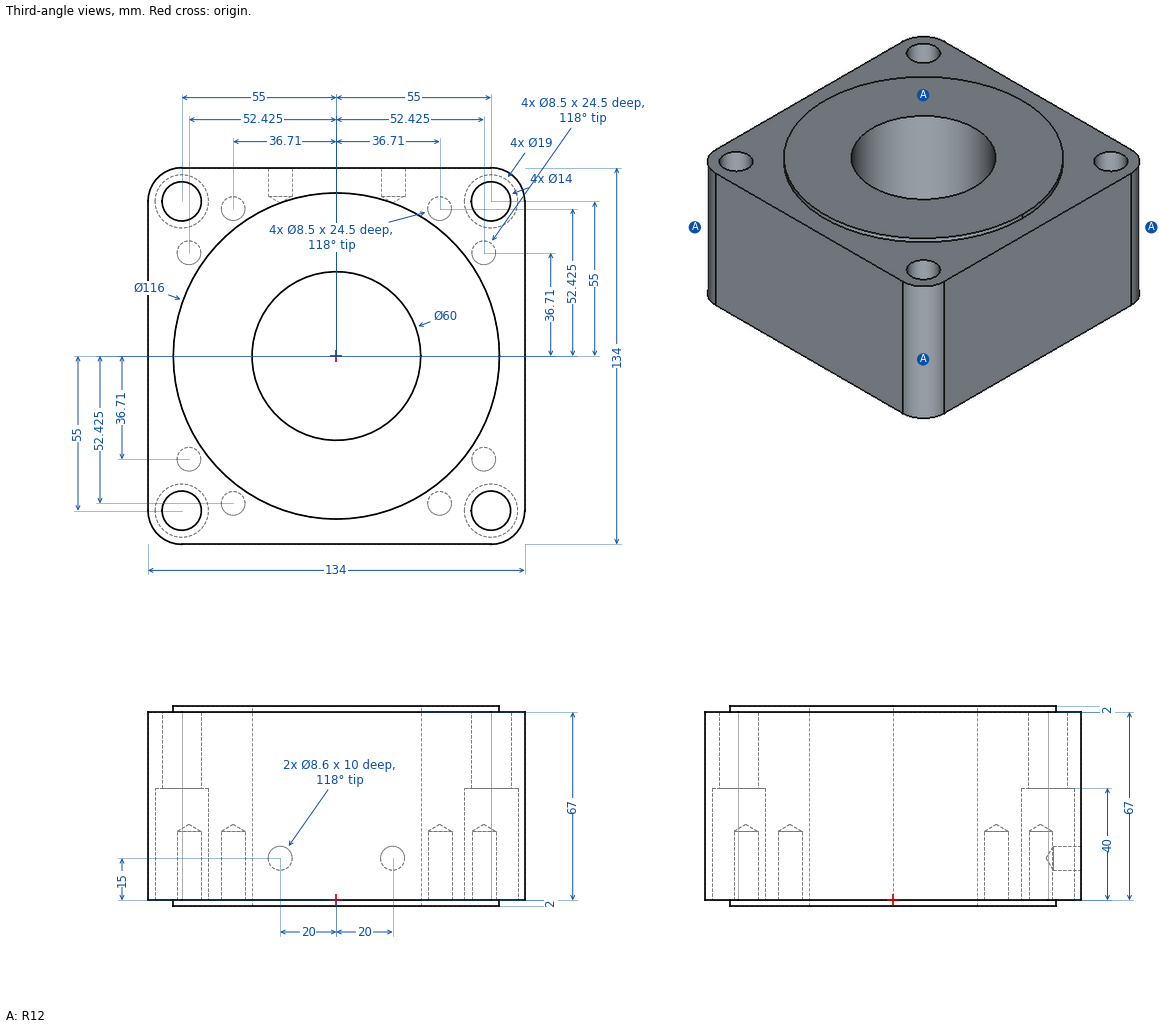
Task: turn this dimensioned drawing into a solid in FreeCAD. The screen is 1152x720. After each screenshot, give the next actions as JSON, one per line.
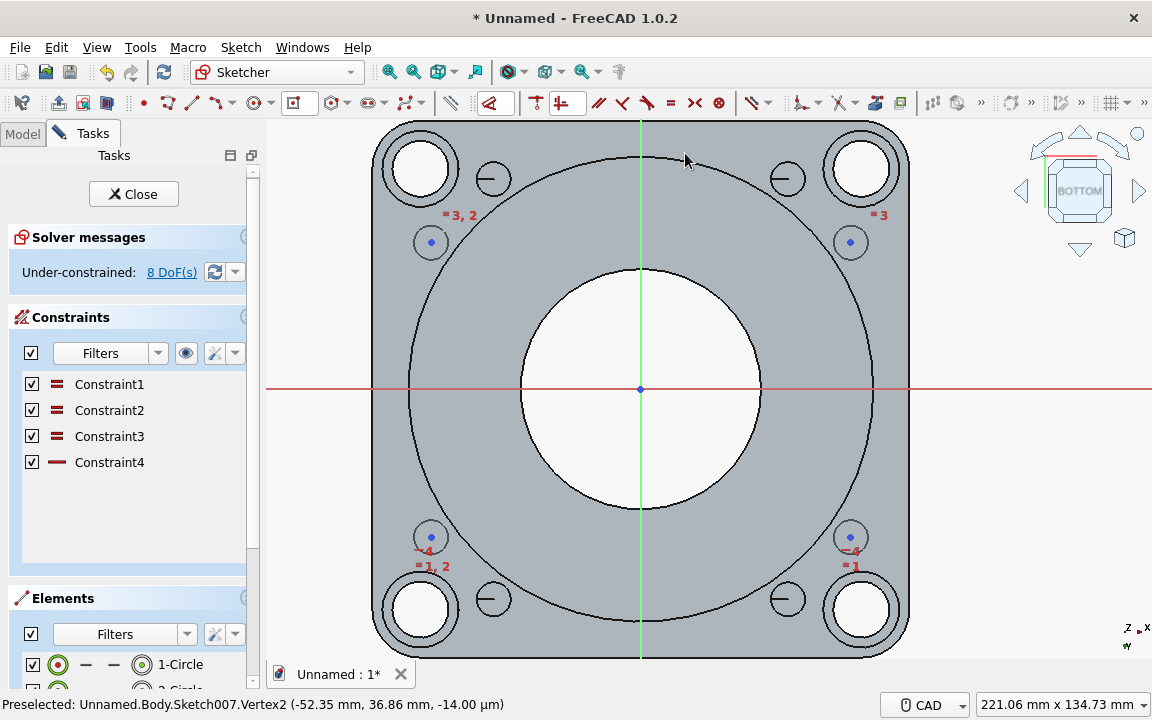
{"action": "left_click", "coordinate": [431, 537]}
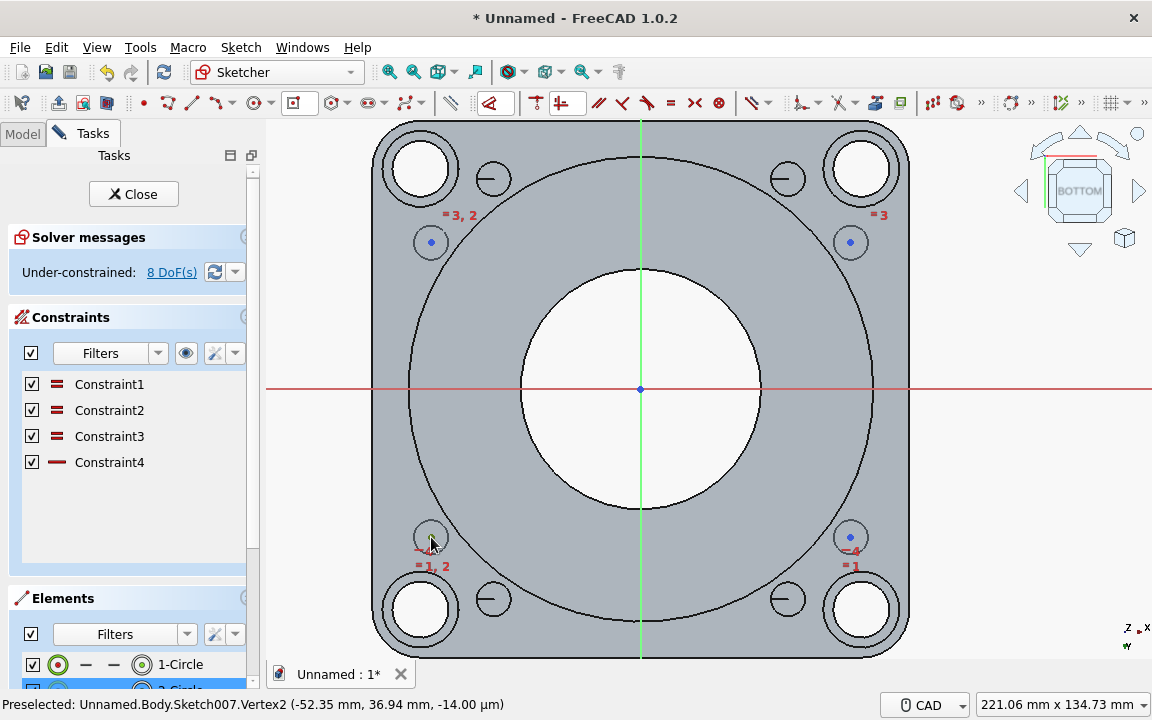
{"action": "left_click", "coordinate": [431, 243]}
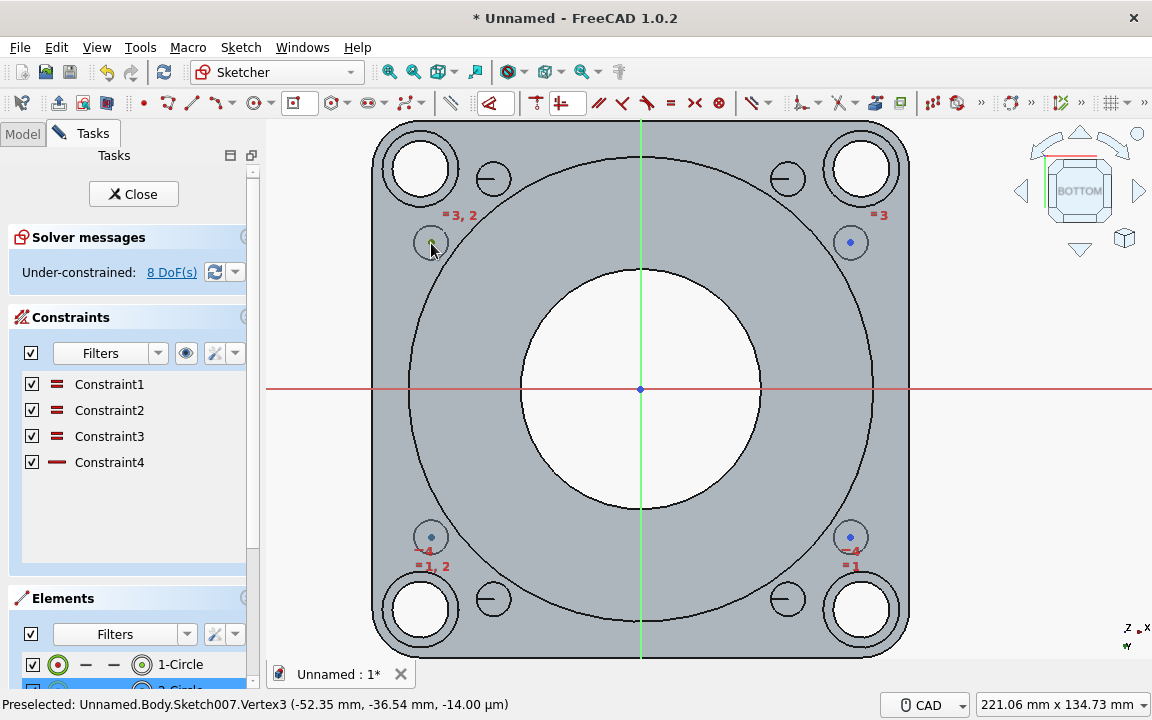
{"action": "left_click", "coordinate": [580, 104]}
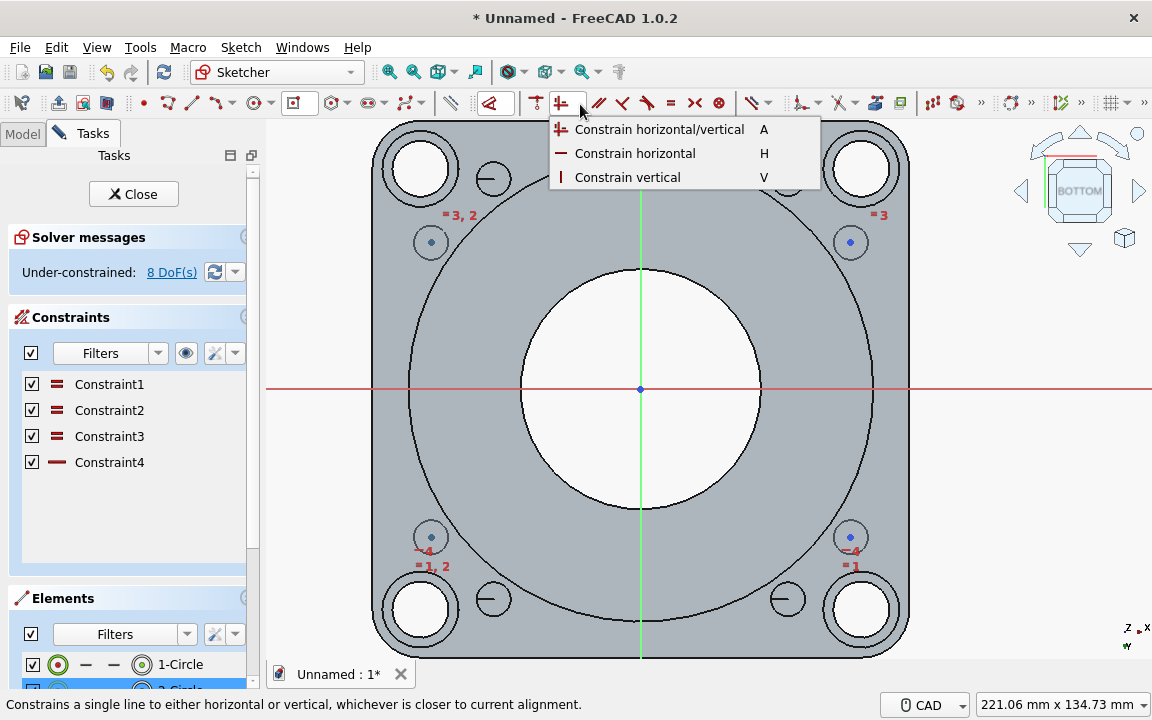
{"action": "left_click", "coordinate": [685, 177]}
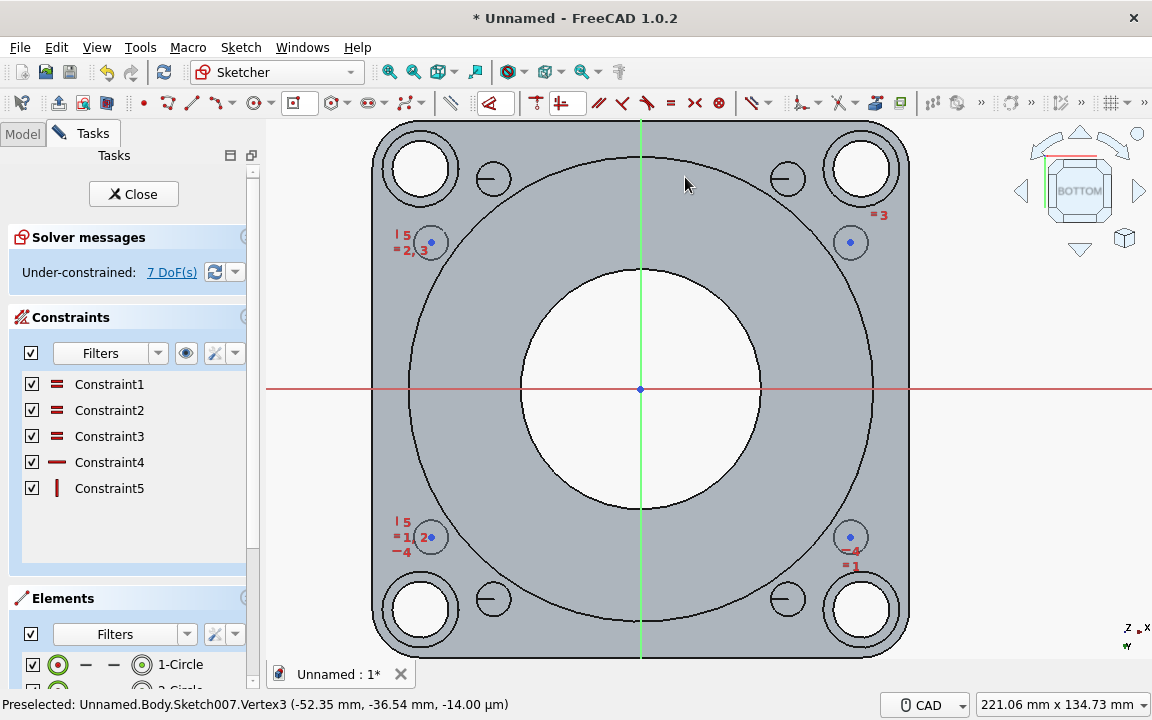
{"action": "left_click", "coordinate": [851, 537]}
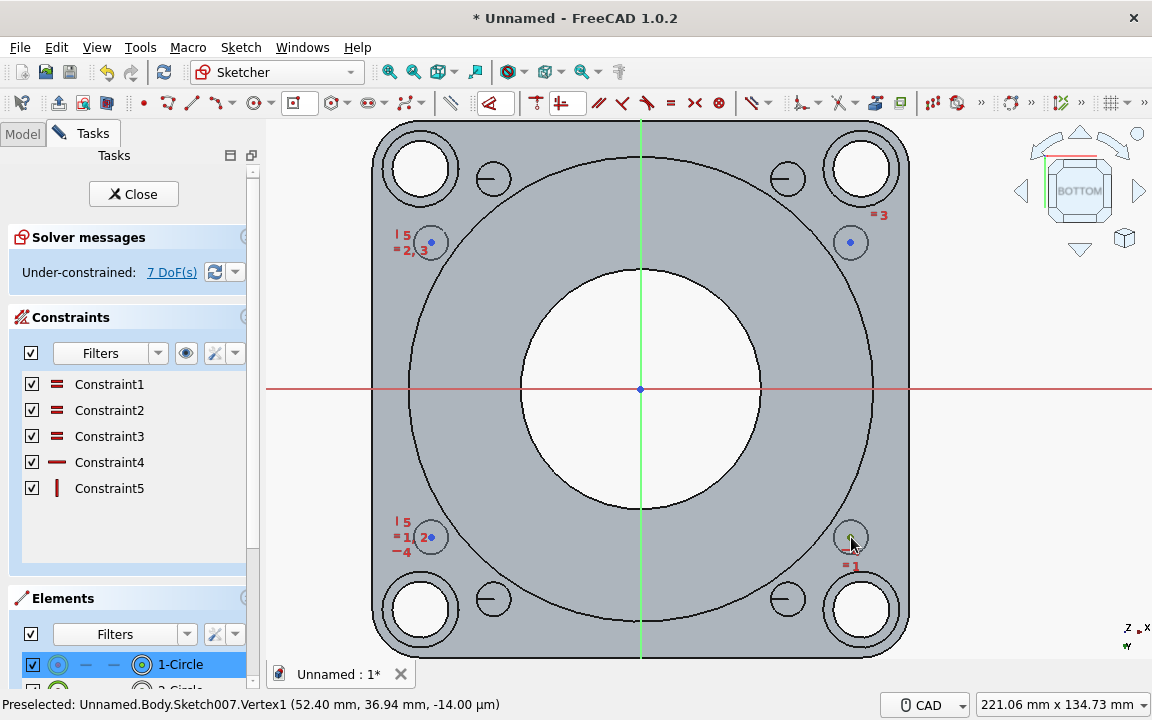
{"action": "left_click", "coordinate": [851, 243]}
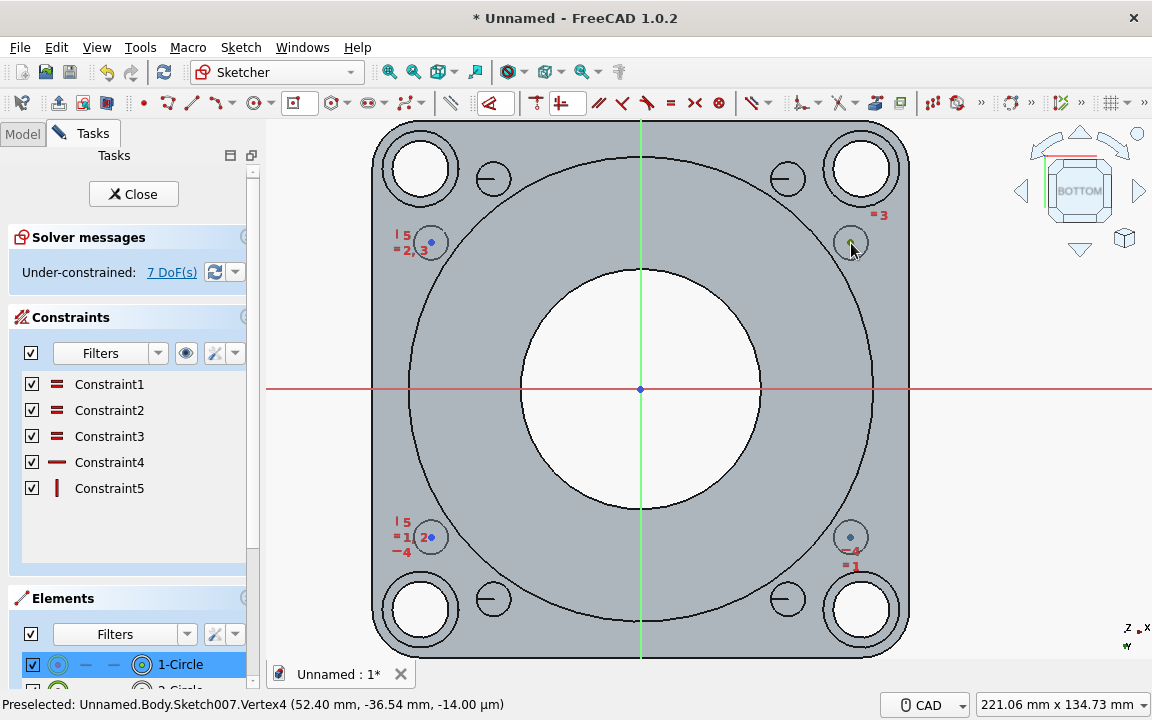
{"action": "key", "text": "v"}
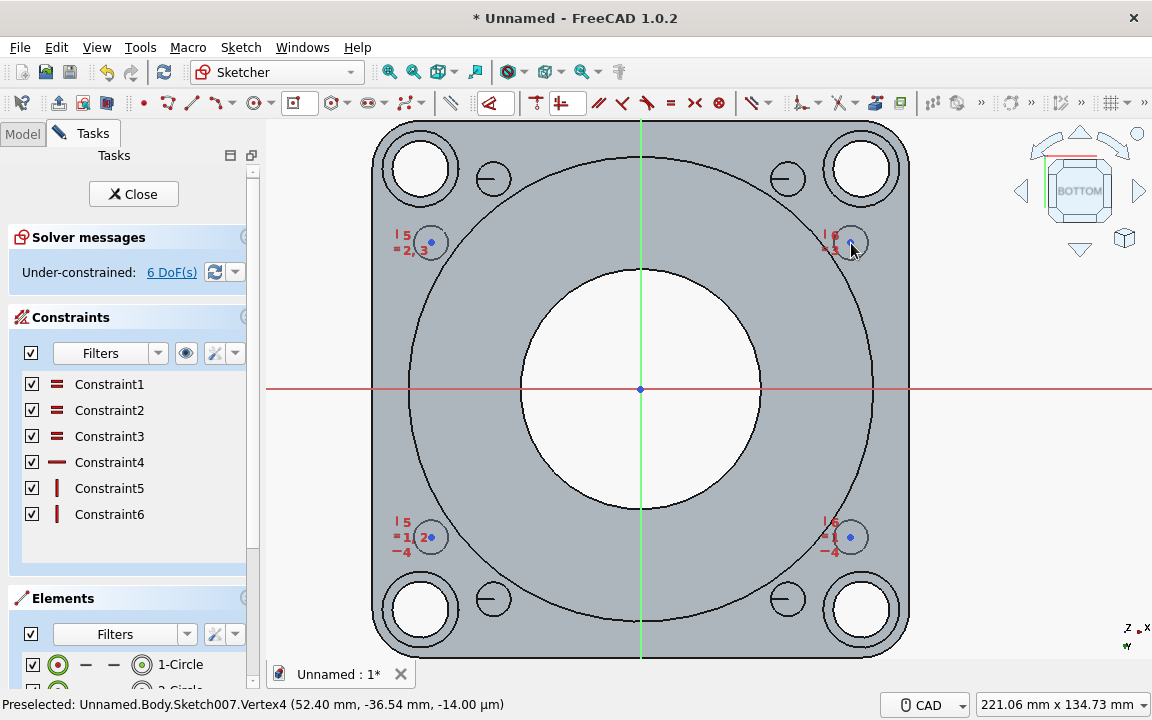
{"action": "left_click", "coordinate": [431, 243]}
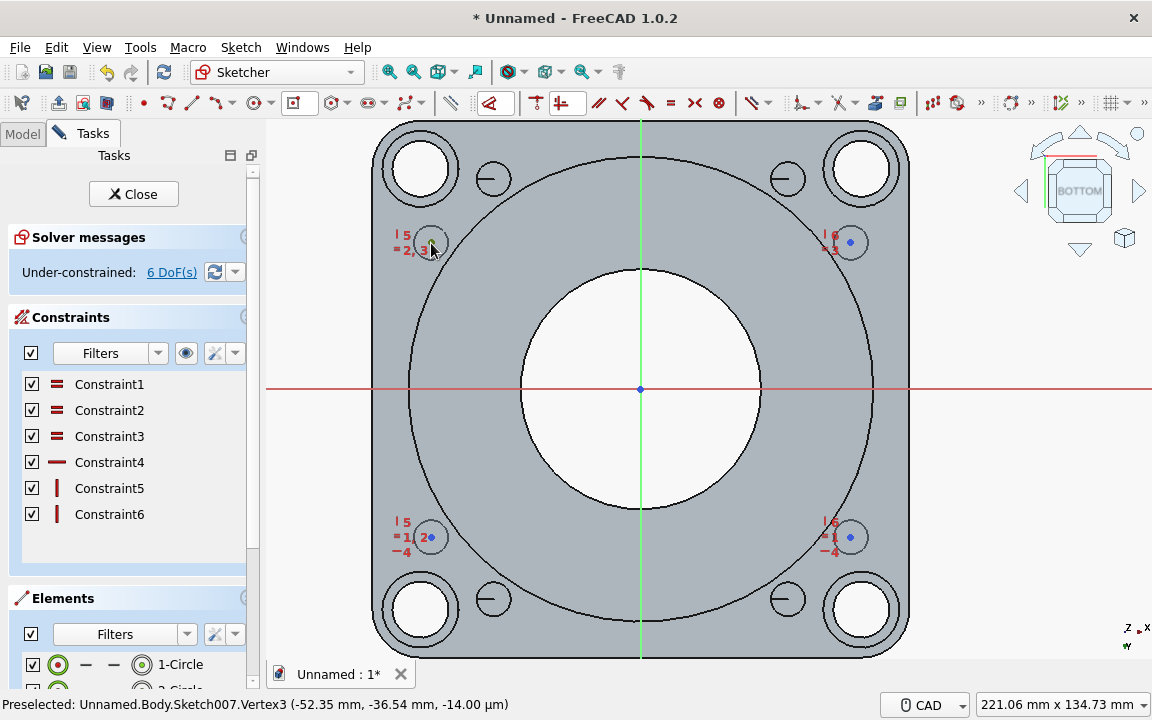
{"action": "left_click", "coordinate": [851, 243]}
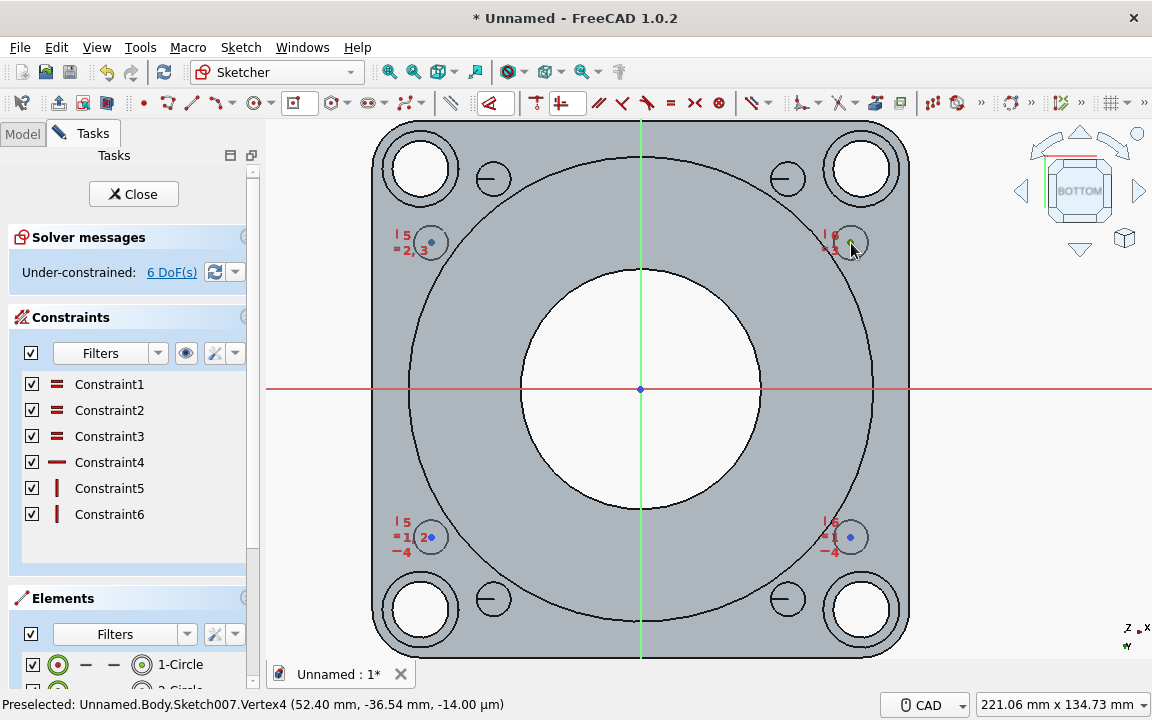
{"action": "left_click", "coordinate": [580, 104]}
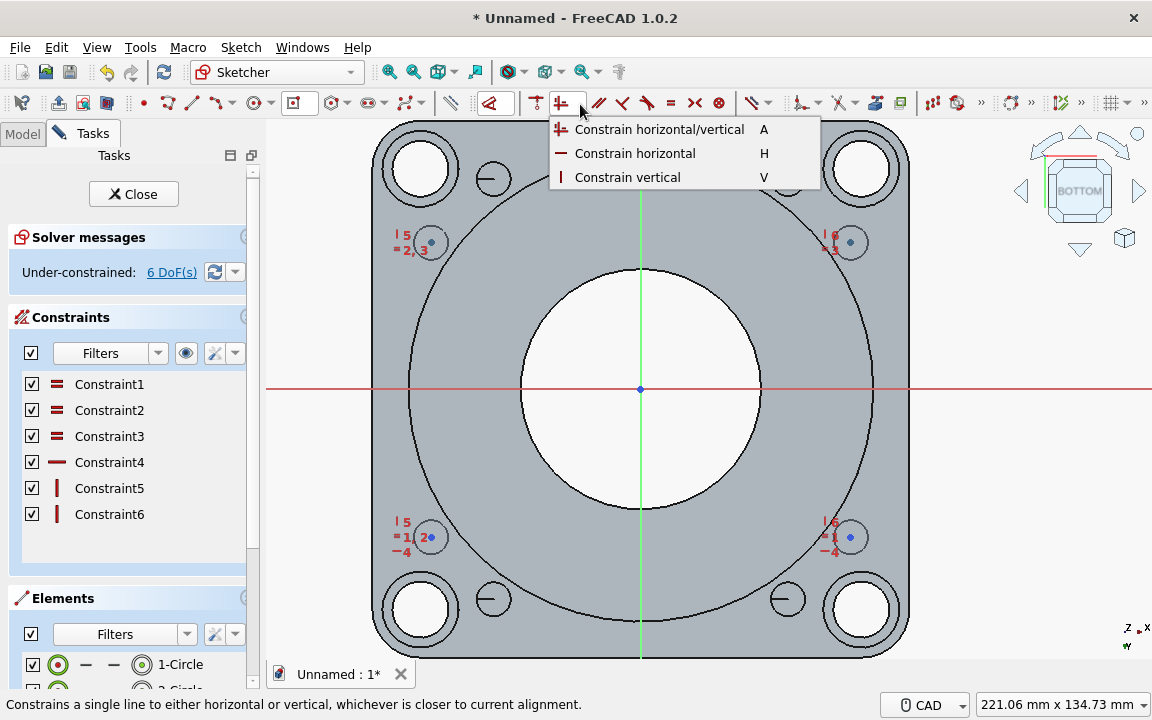
{"action": "left_click", "coordinate": [685, 153]}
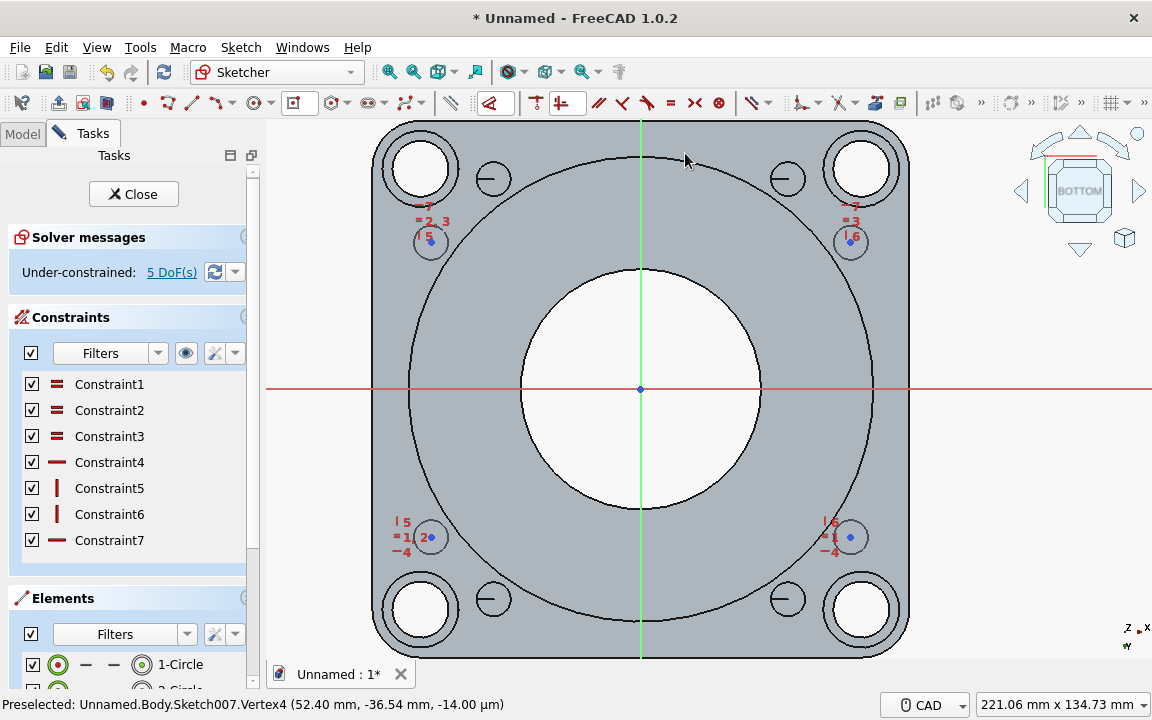
{"action": "left_click", "coordinate": [863, 525]}